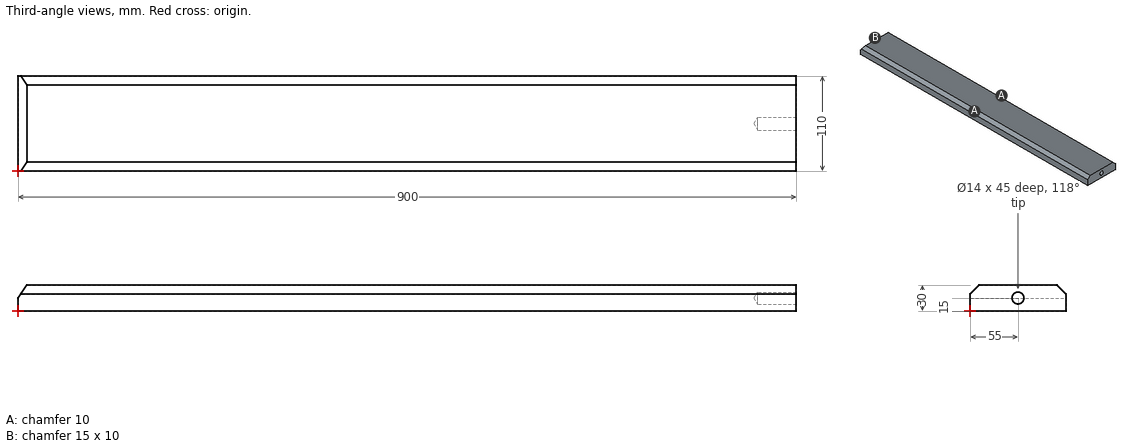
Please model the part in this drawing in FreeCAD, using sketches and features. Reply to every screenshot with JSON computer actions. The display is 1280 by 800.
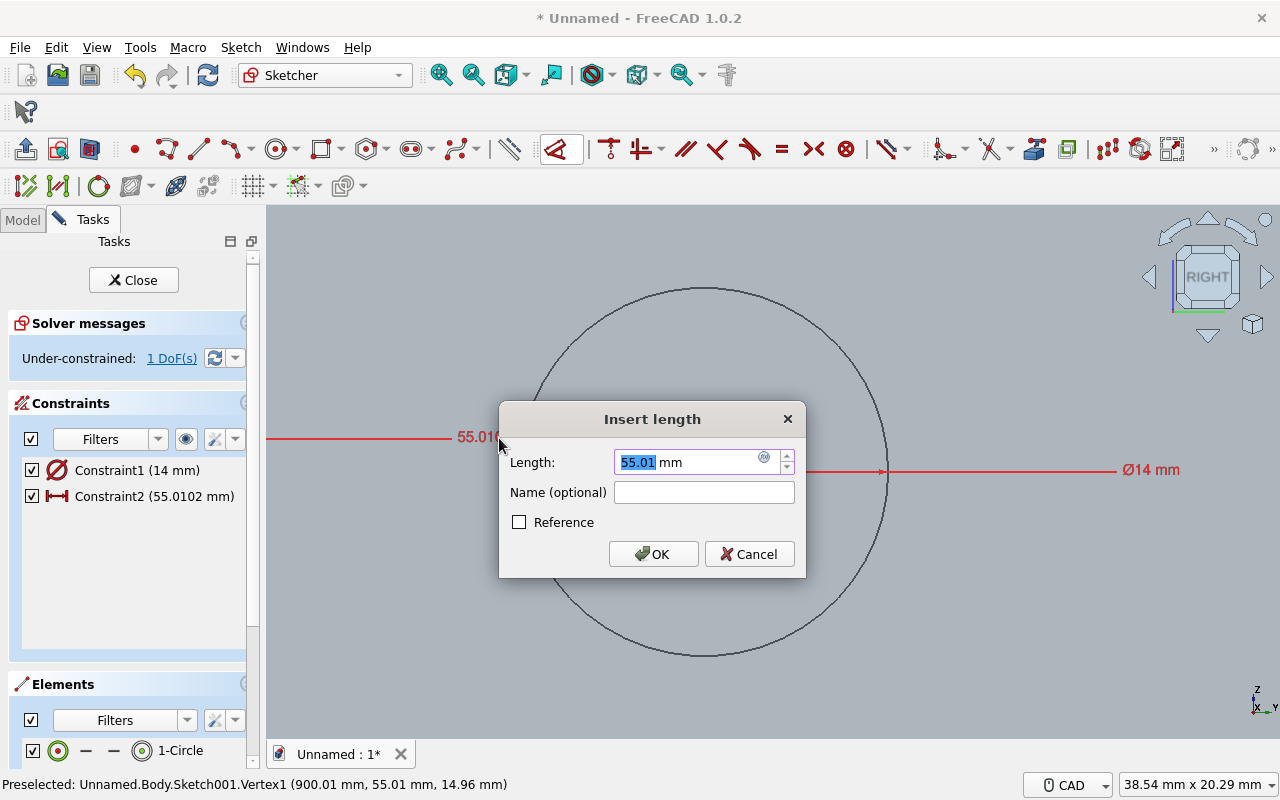
{"action": "type", "text": "55"}
{"action": "key", "text": "Return"}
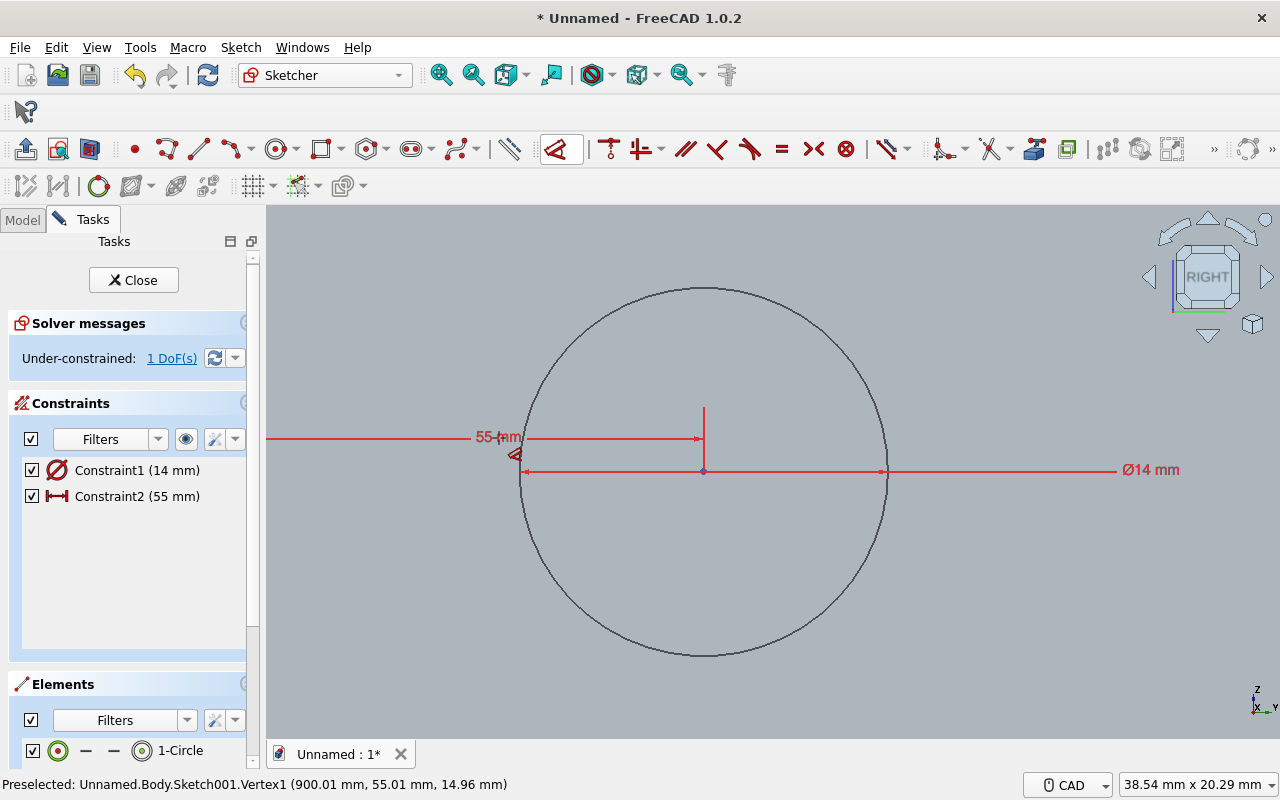
{"action": "left_click", "coordinate": [704, 472]}
{"action": "left_click", "coordinate": [738, 591]}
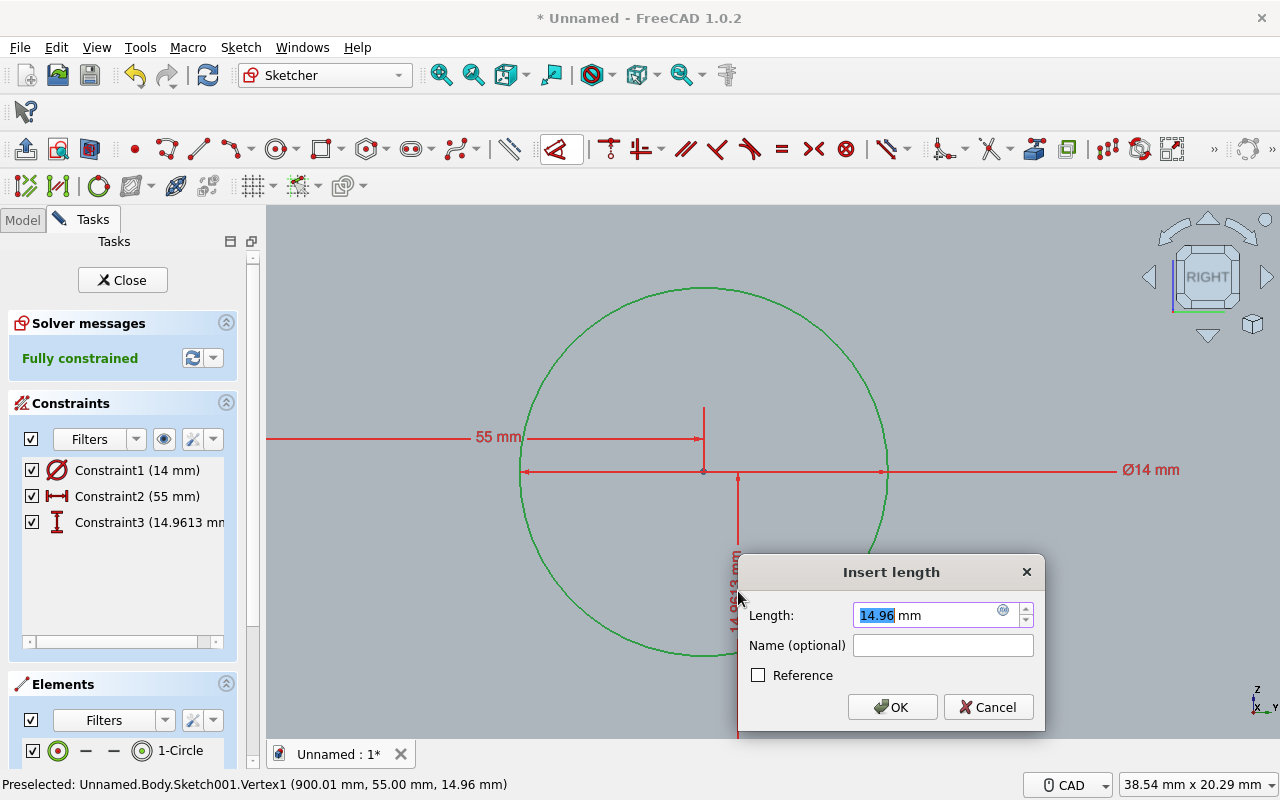
{"action": "type", "text": "15"}
{"action": "key", "text": "Return"}
{"action": "key", "text": "Escape"}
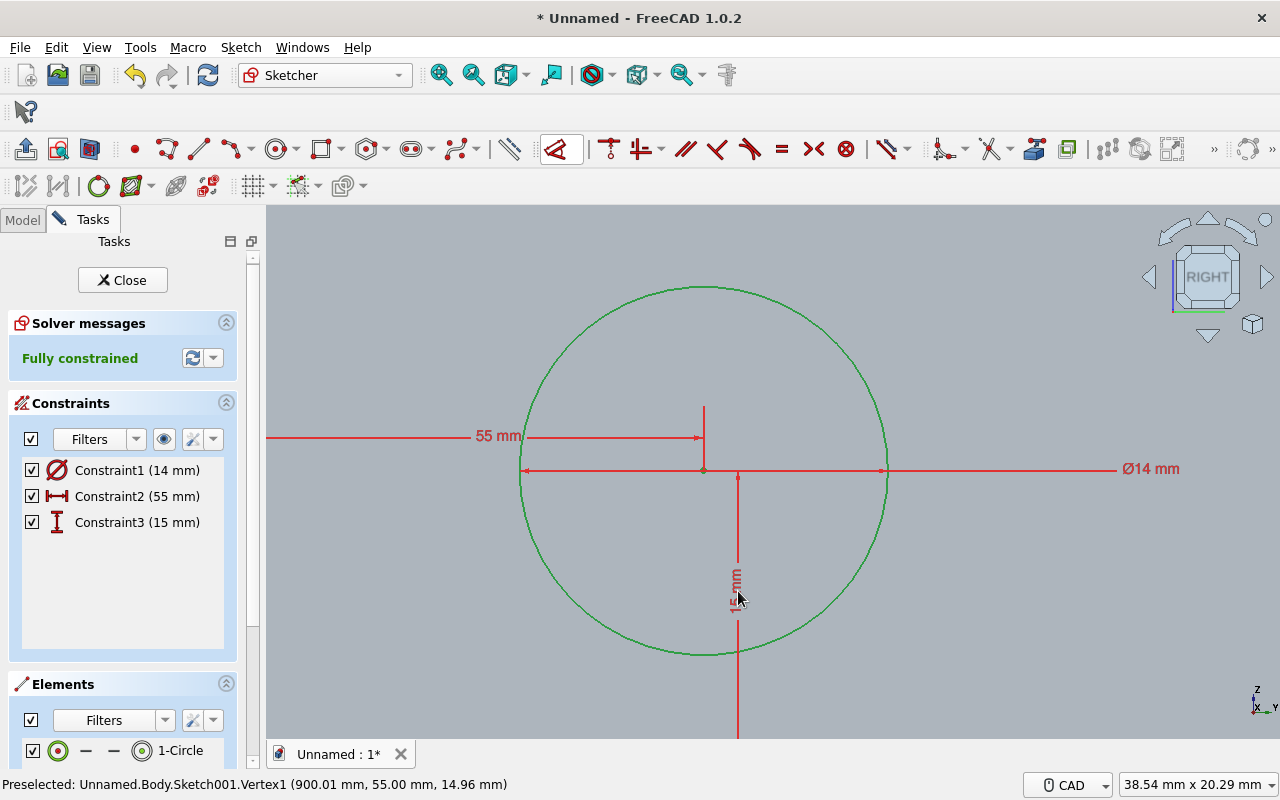
{"action": "left_click", "coordinate": [123, 280]}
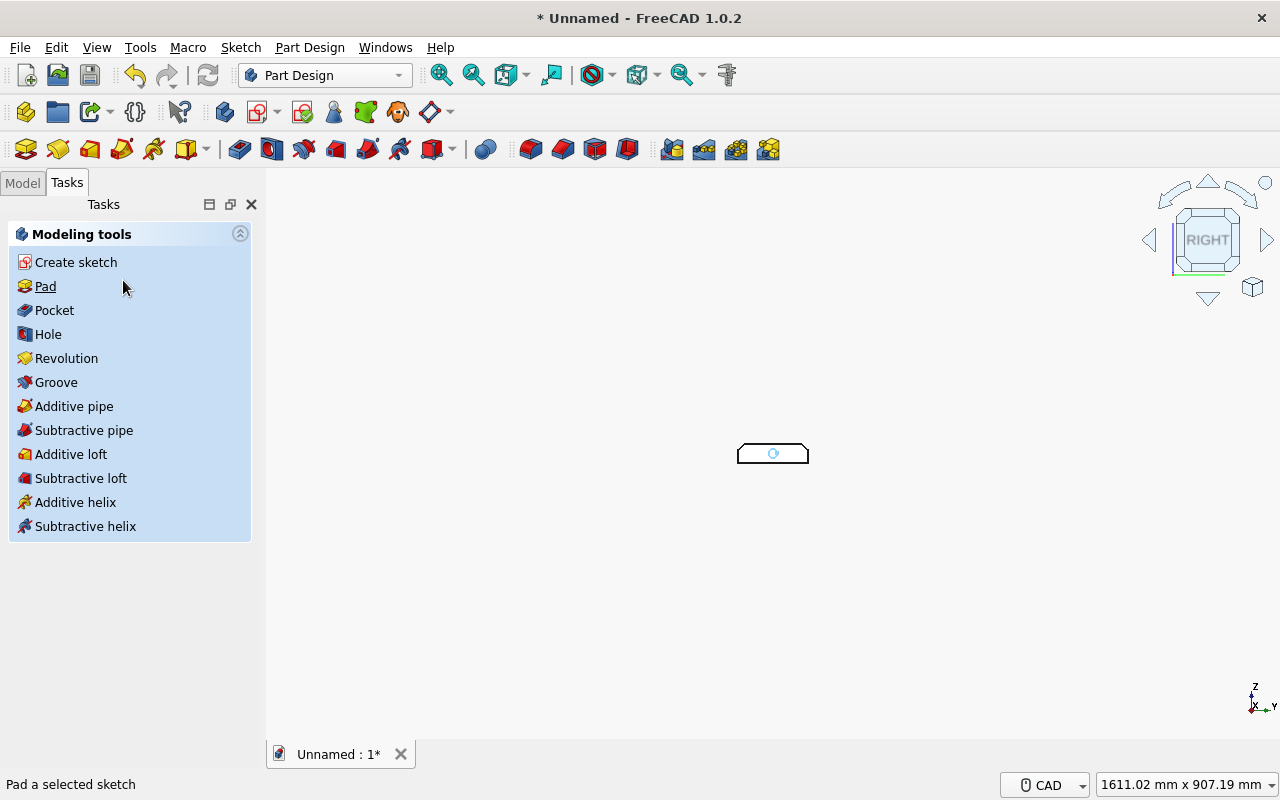
{"action": "left_click", "coordinate": [272, 150]}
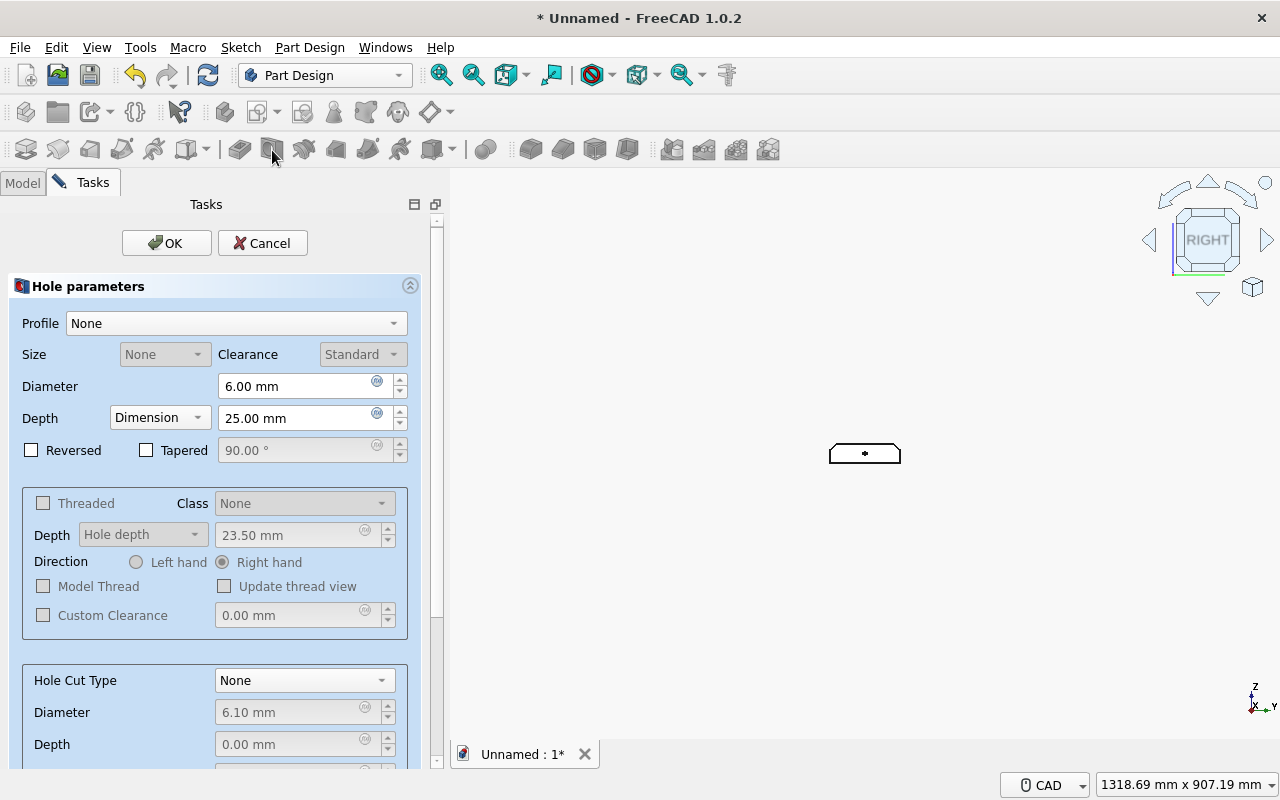
{"action": "triple_click", "coordinate": [305, 386]}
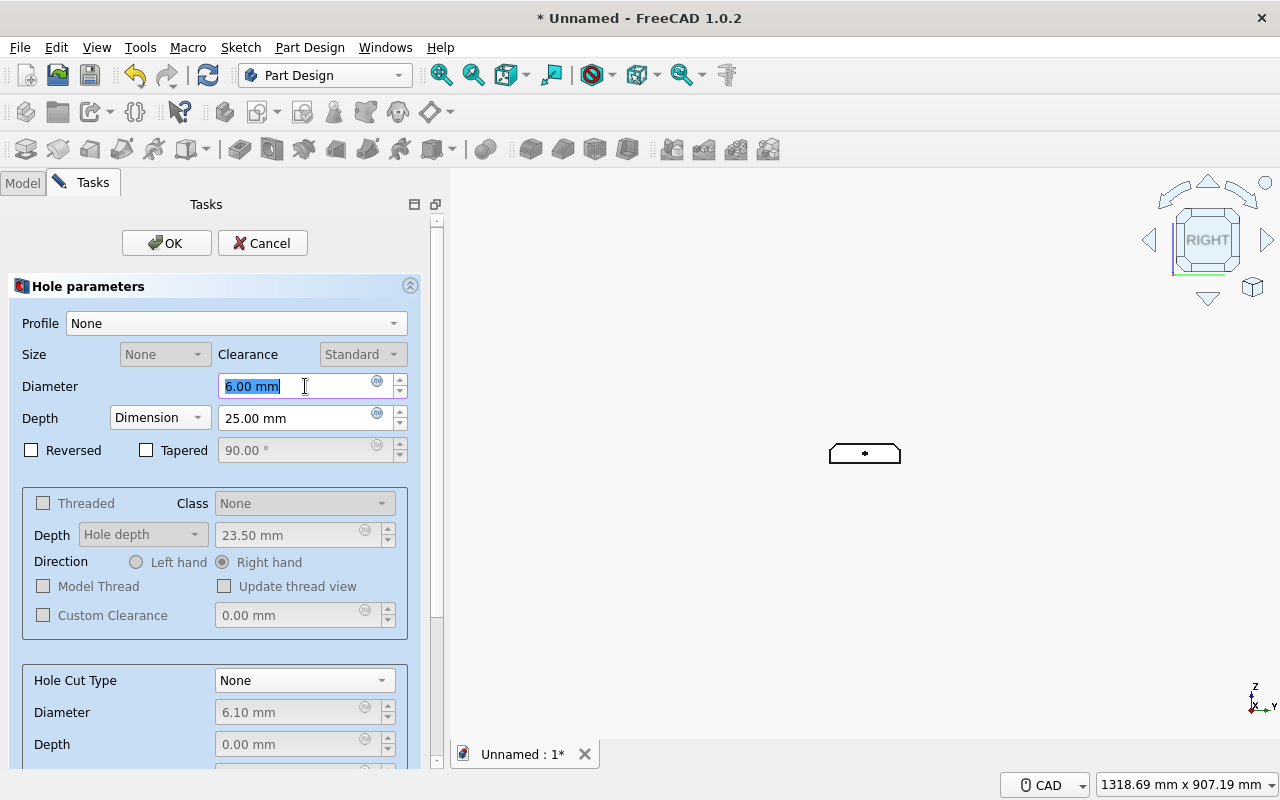
{"action": "type", "text": "14"}
{"action": "key", "text": "Tab"}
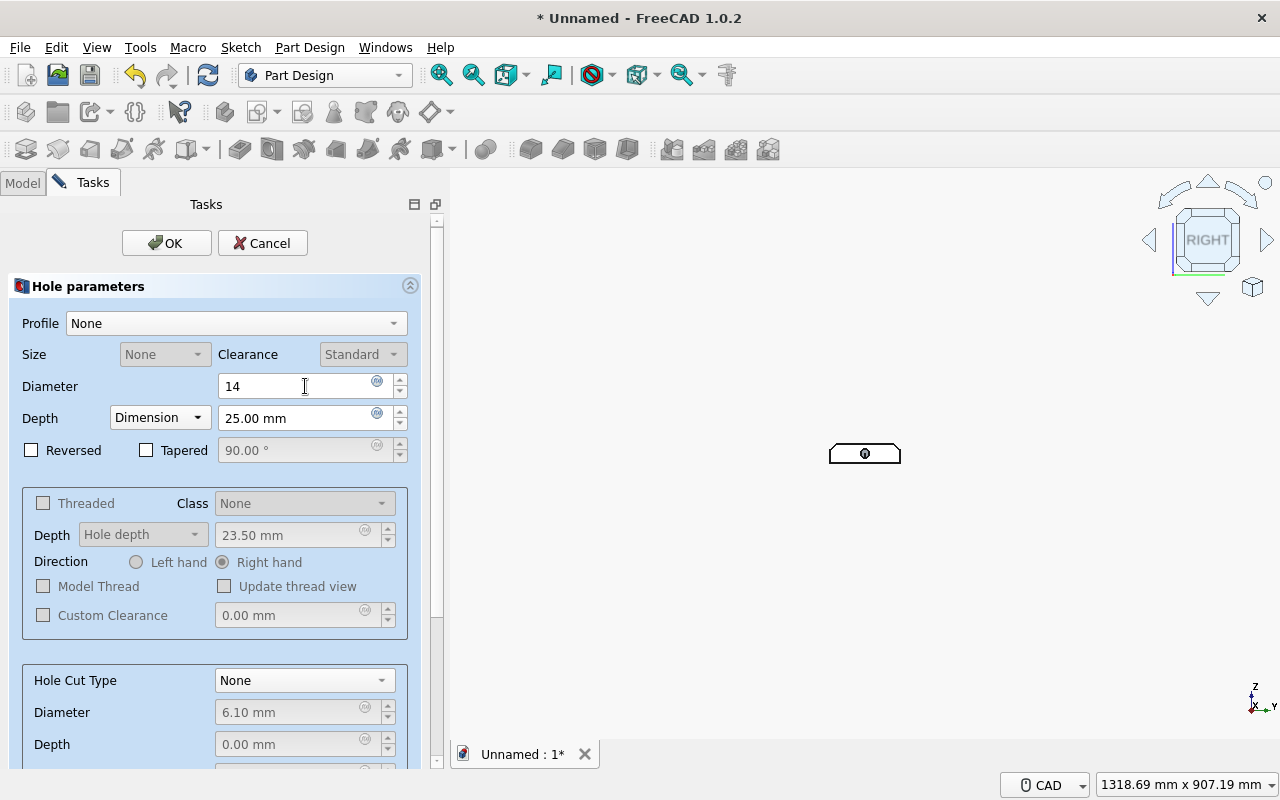
{"action": "triple_click", "coordinate": [305, 418]}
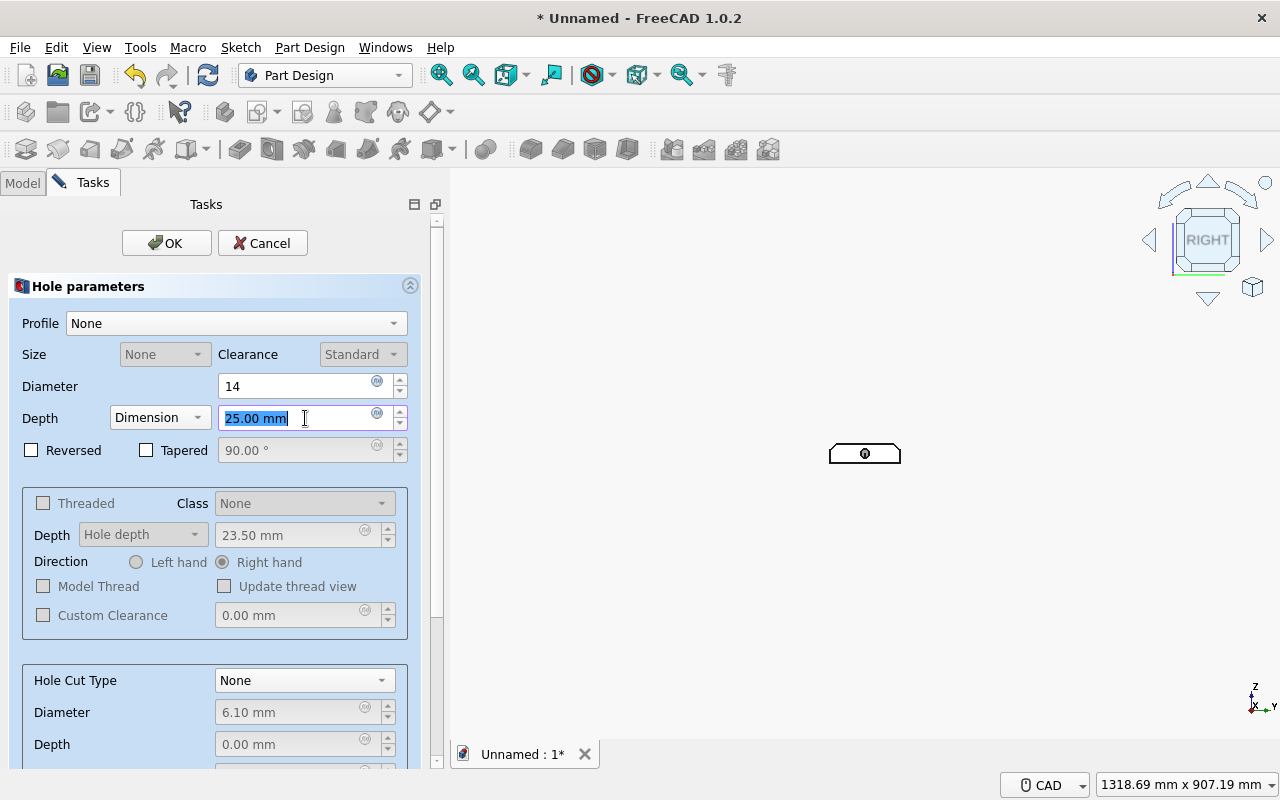
{"action": "type", "text": "45"}
{"action": "key", "text": "Tab"}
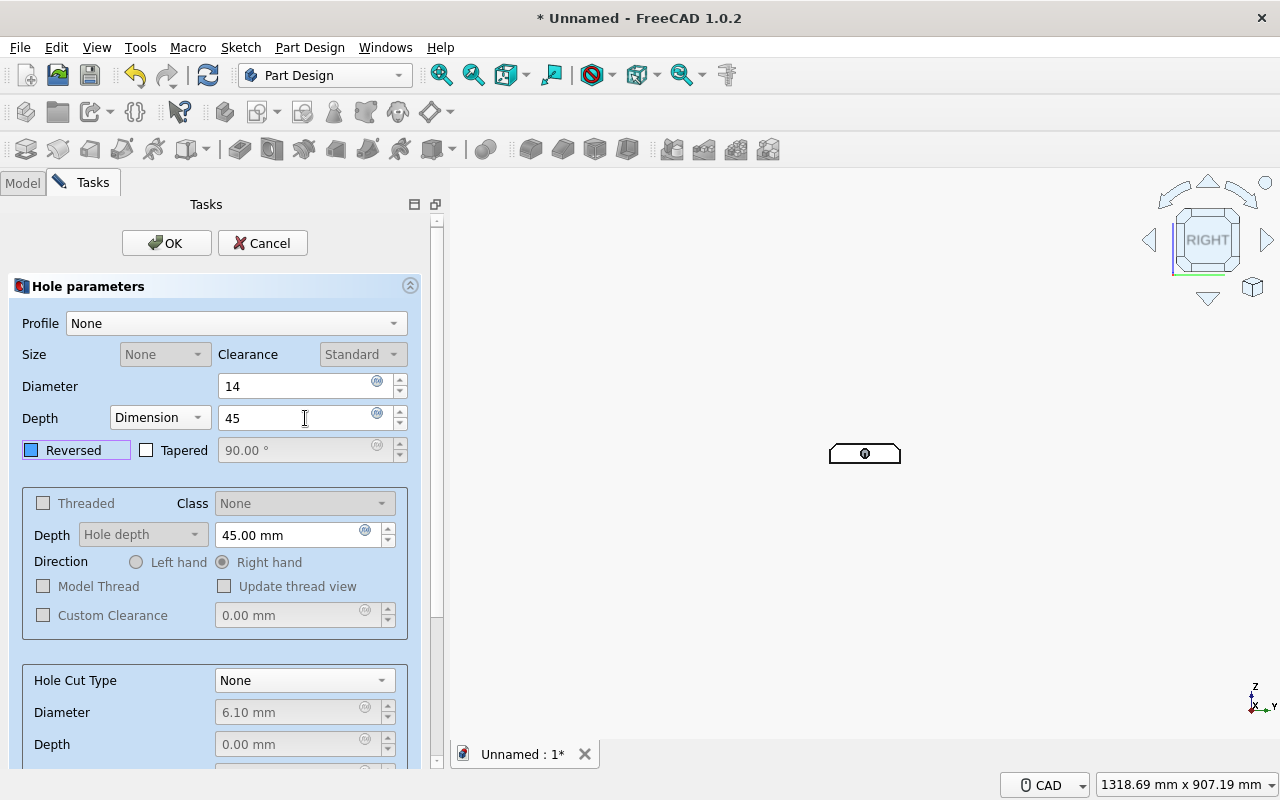
{"action": "left_click", "coordinate": [167, 243]}